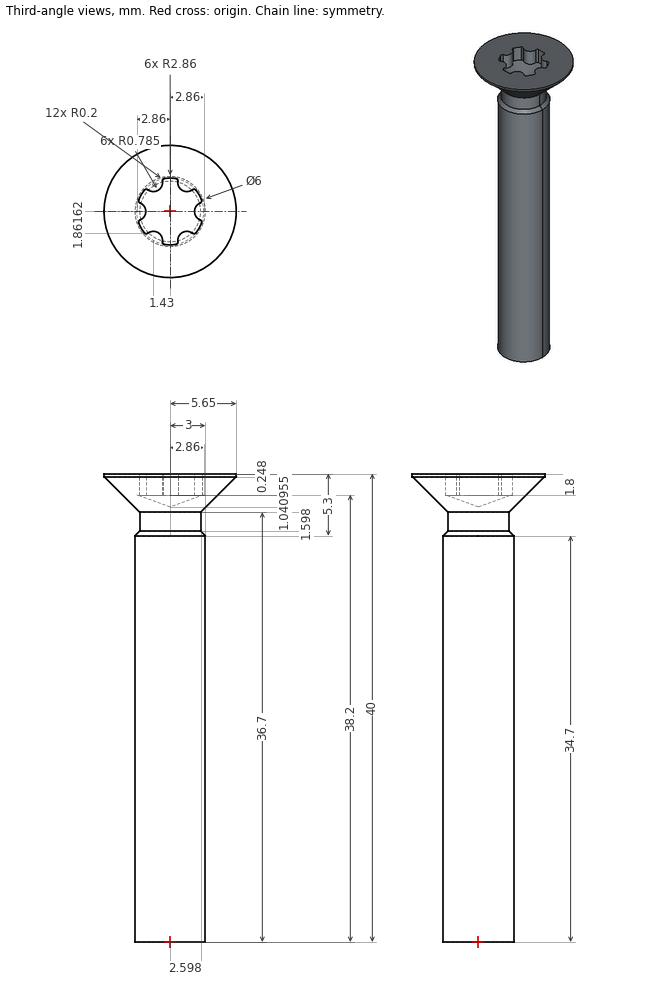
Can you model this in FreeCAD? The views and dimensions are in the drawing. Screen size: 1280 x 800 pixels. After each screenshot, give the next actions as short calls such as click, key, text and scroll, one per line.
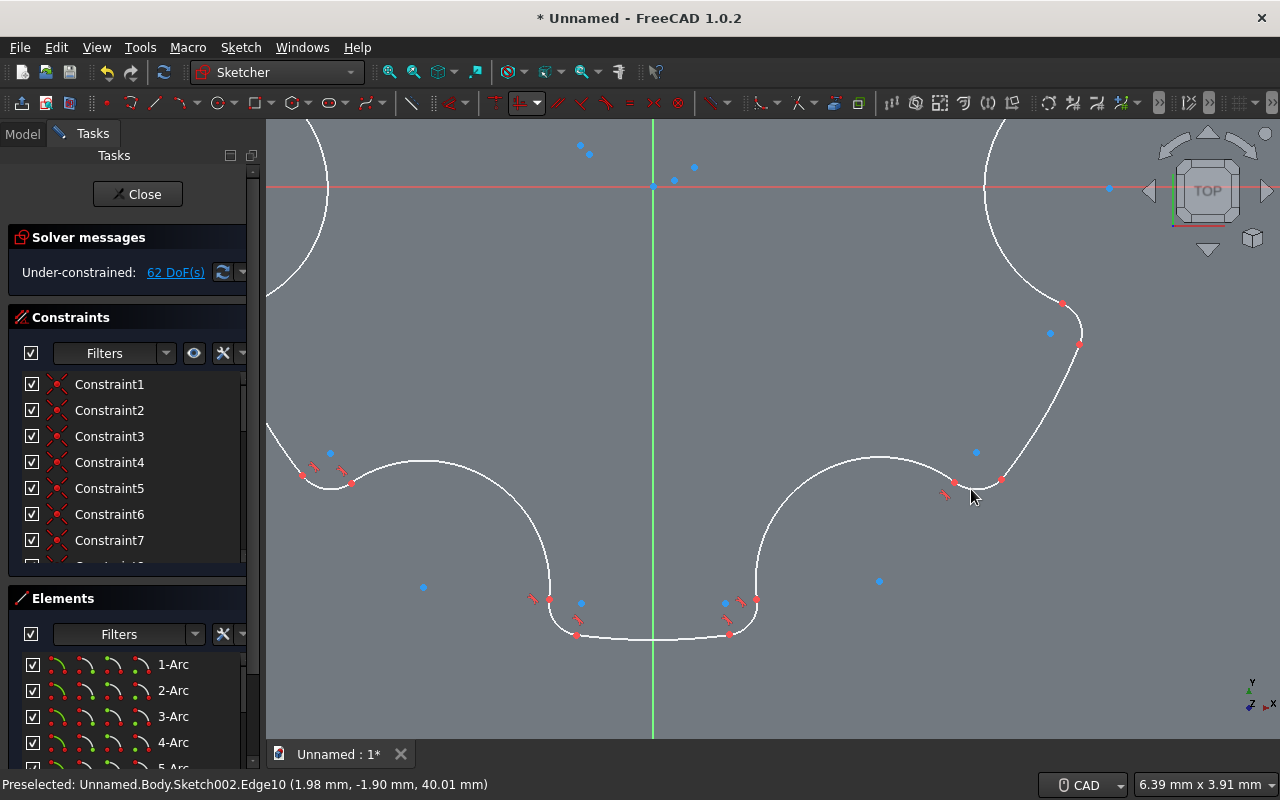
click(968, 488)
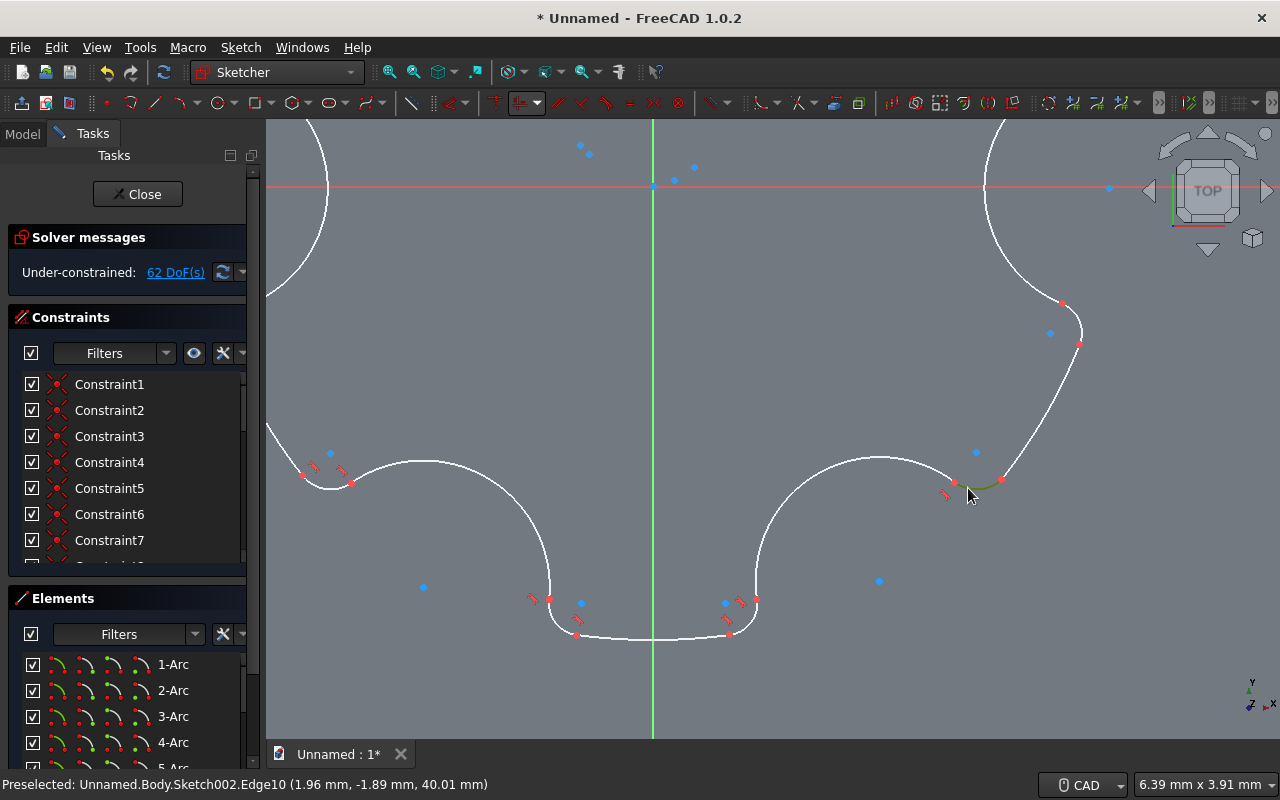
click(1029, 442)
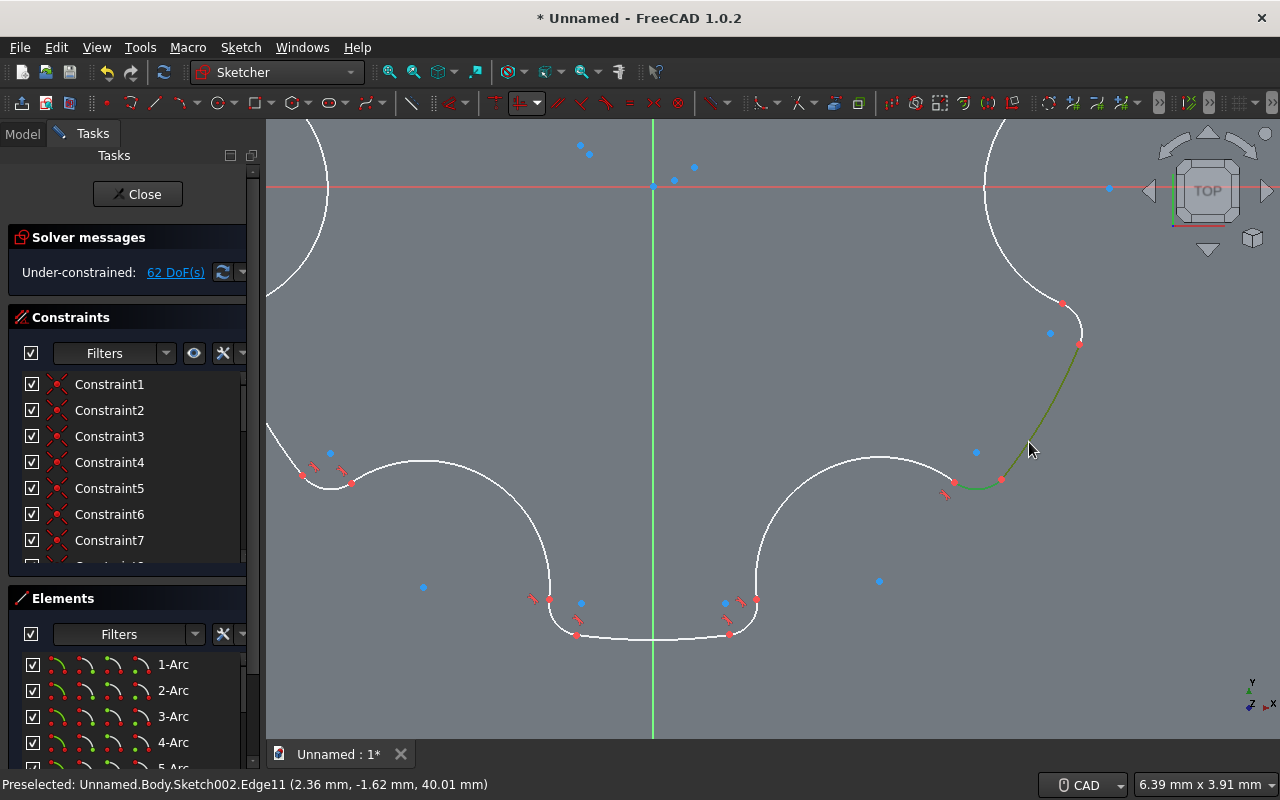
click(606, 104)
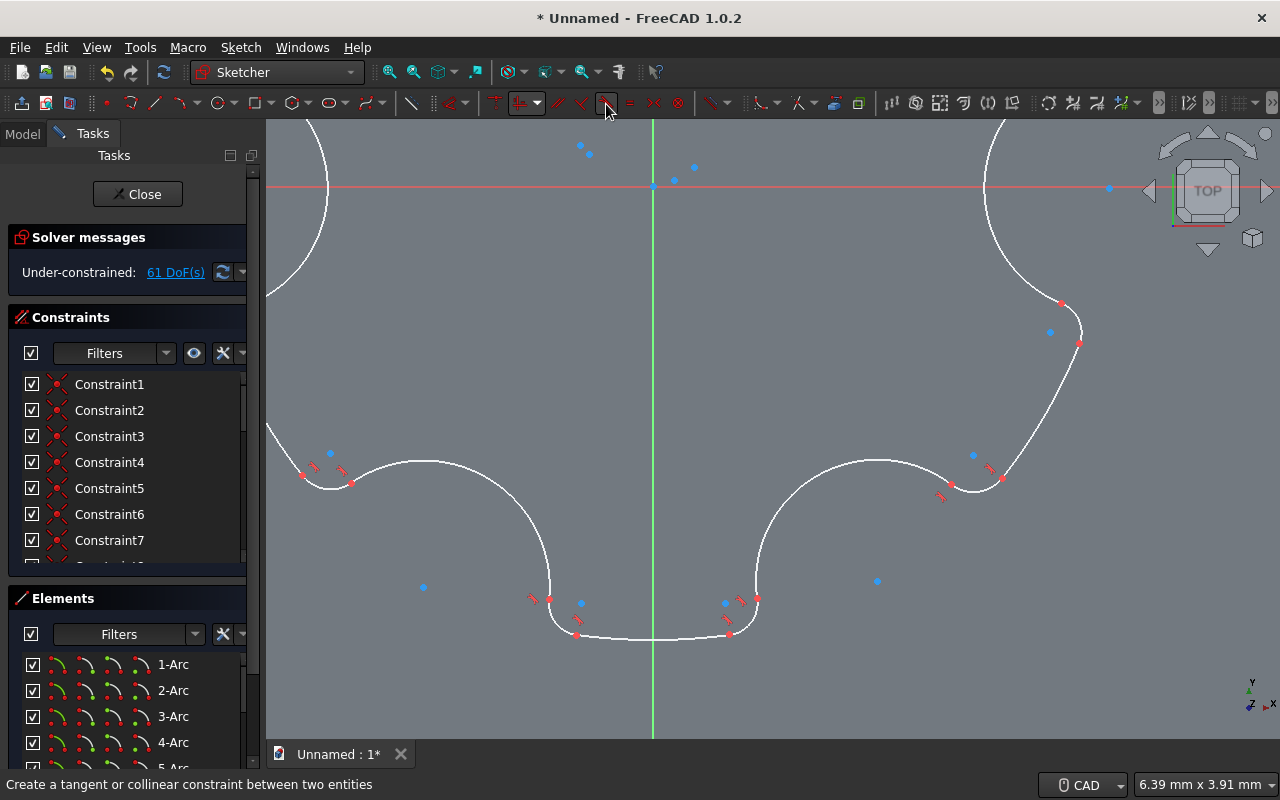
click(1030, 440)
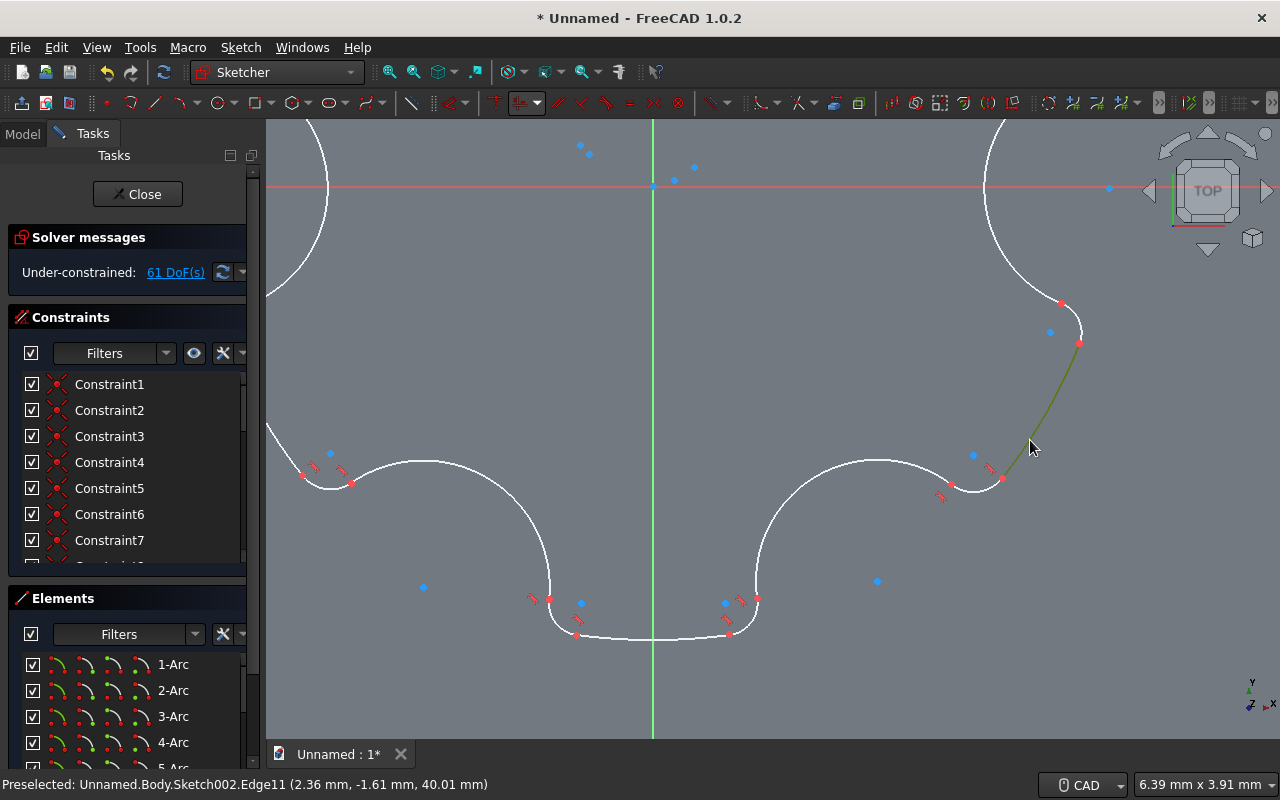
click(1081, 329)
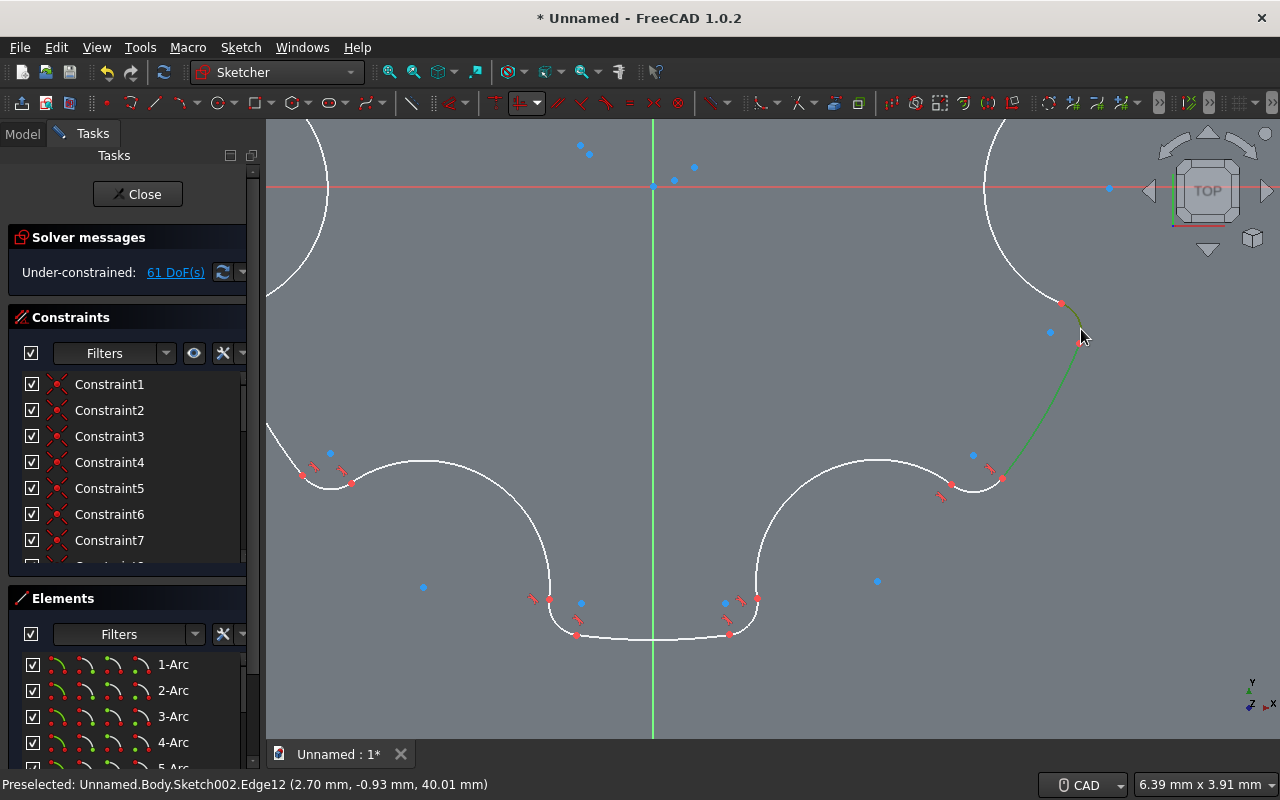
click(606, 104)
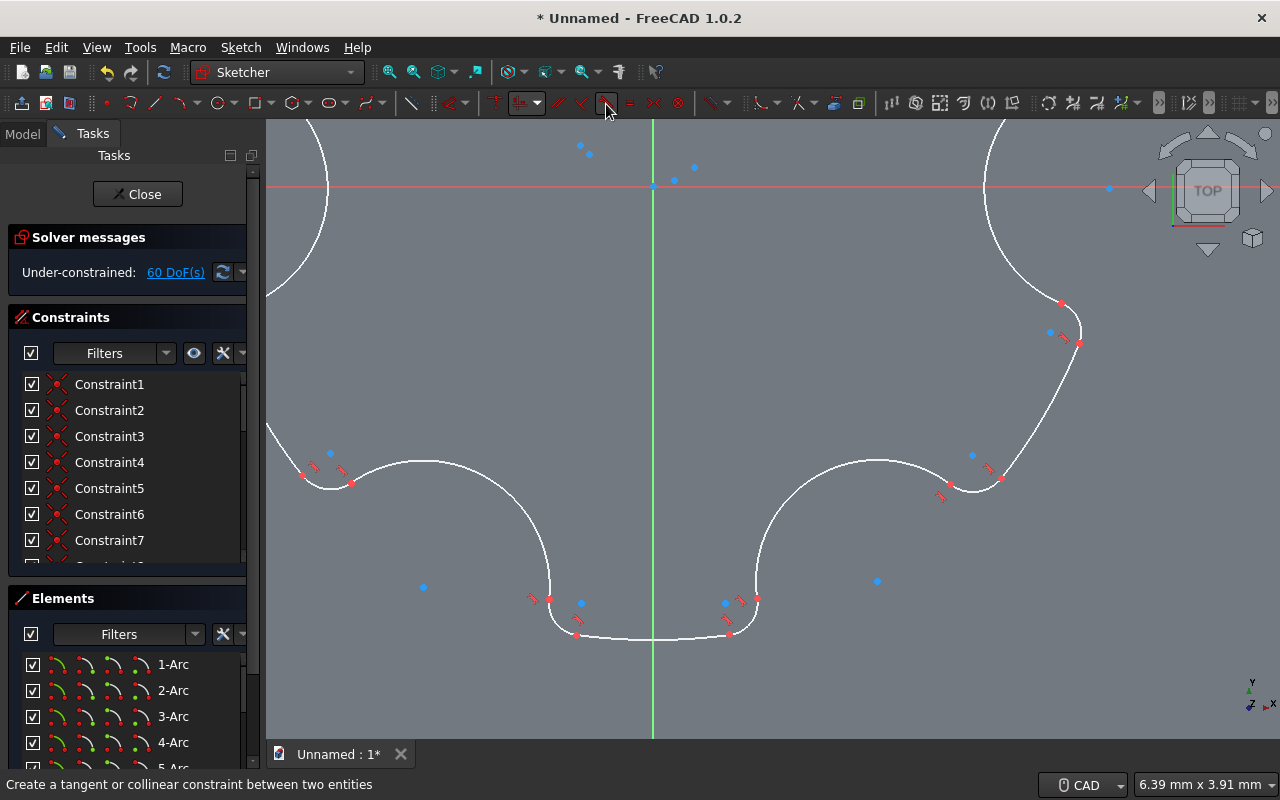
click(1081, 329)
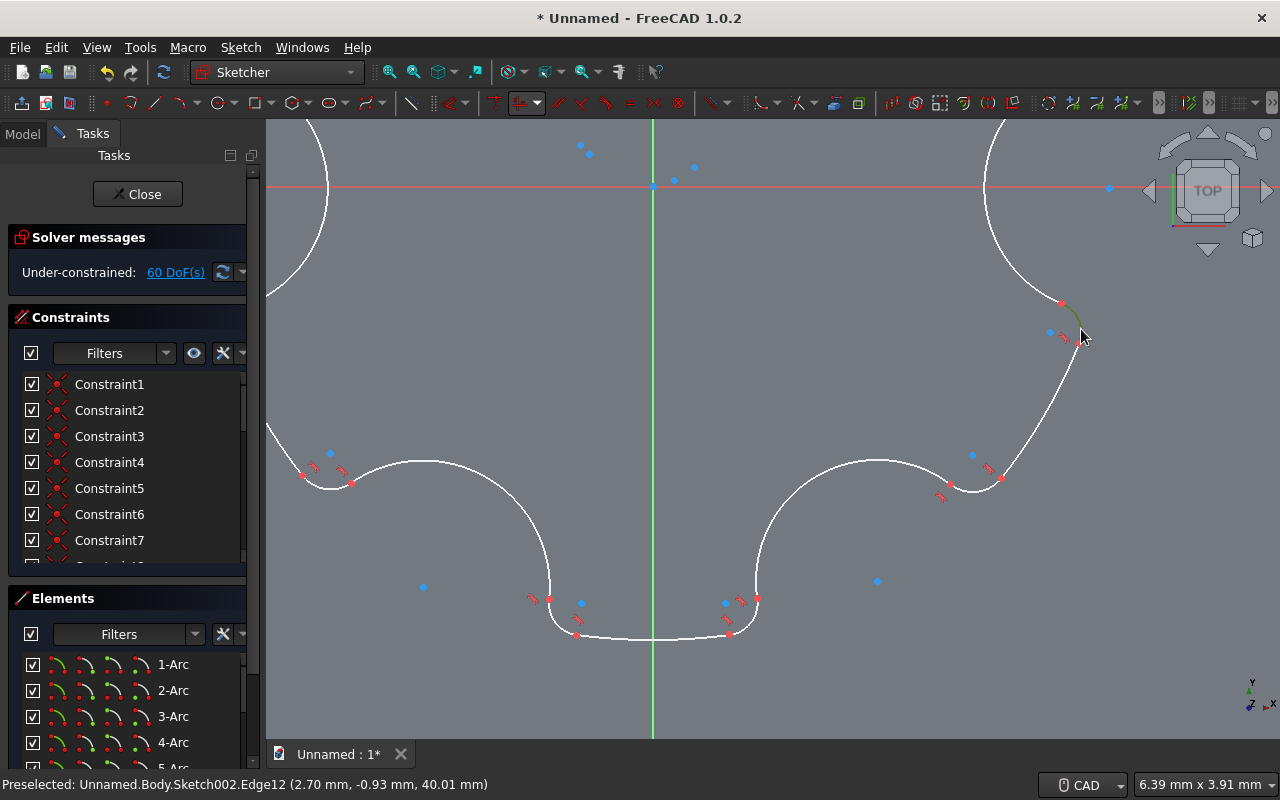
click(998, 245)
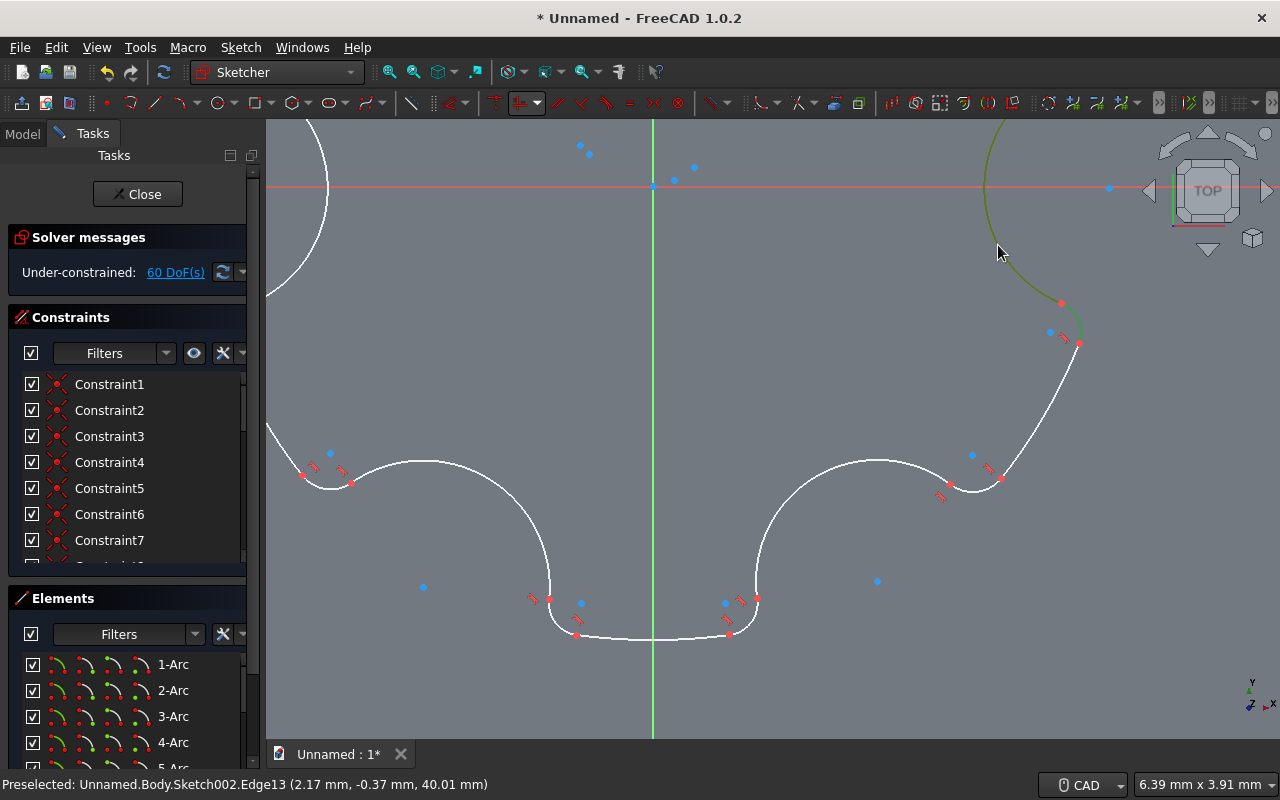
click(606, 104)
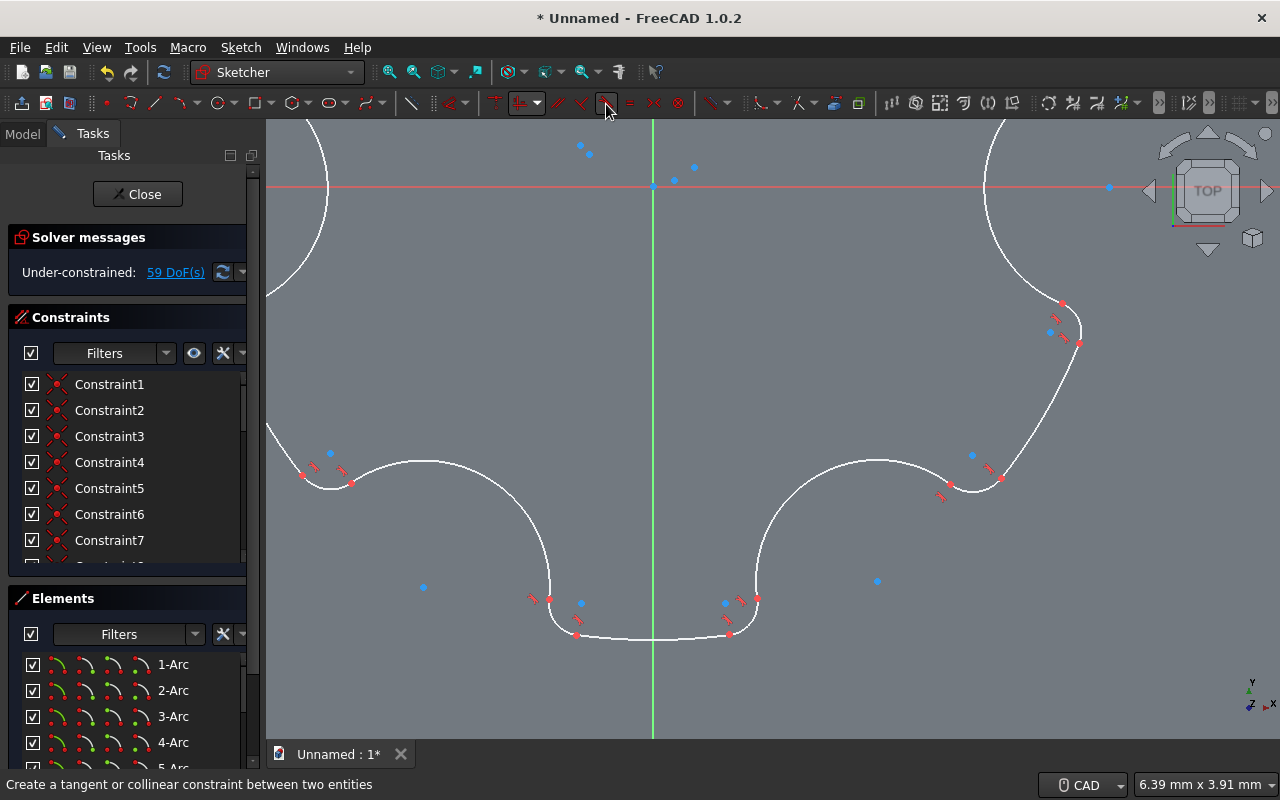
click(998, 245)